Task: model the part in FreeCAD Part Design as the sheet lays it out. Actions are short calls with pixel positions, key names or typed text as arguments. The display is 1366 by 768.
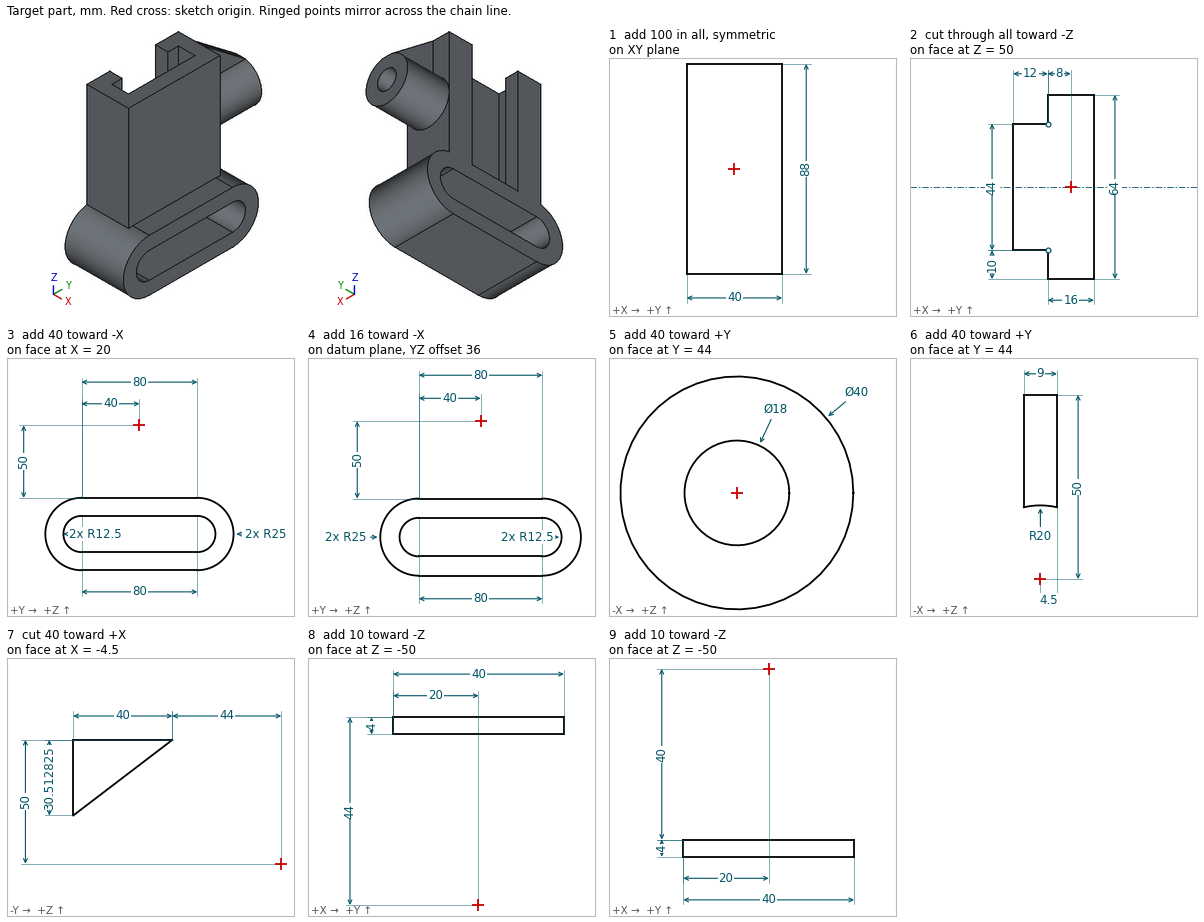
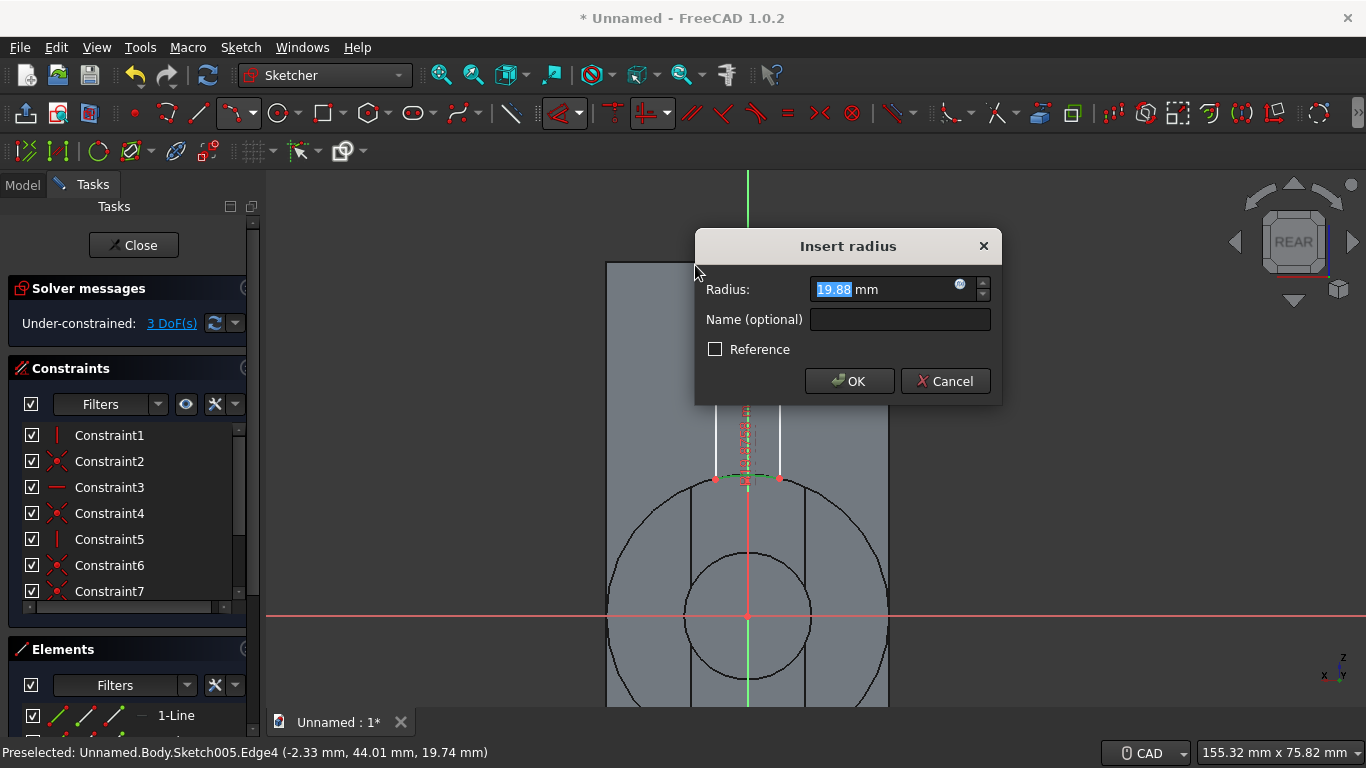
text(20)
key(Return)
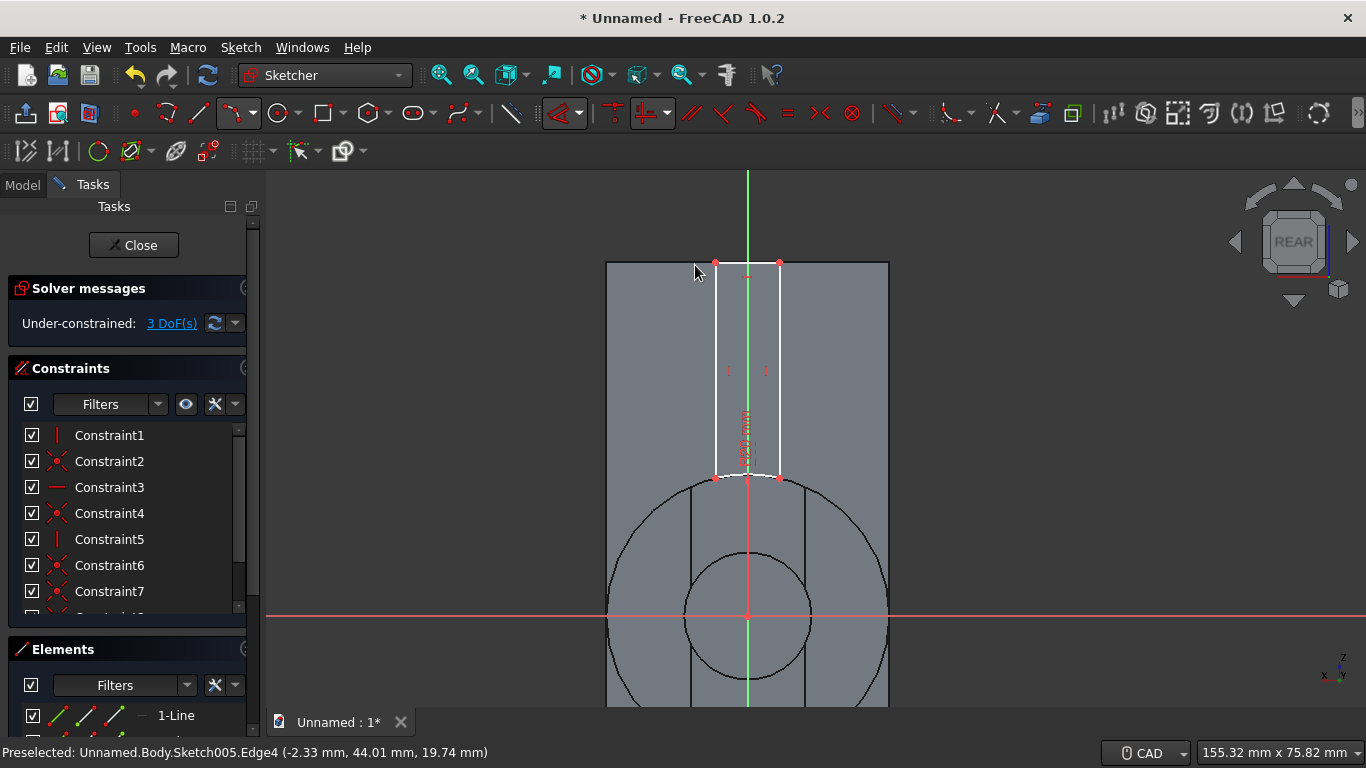
click(760, 263)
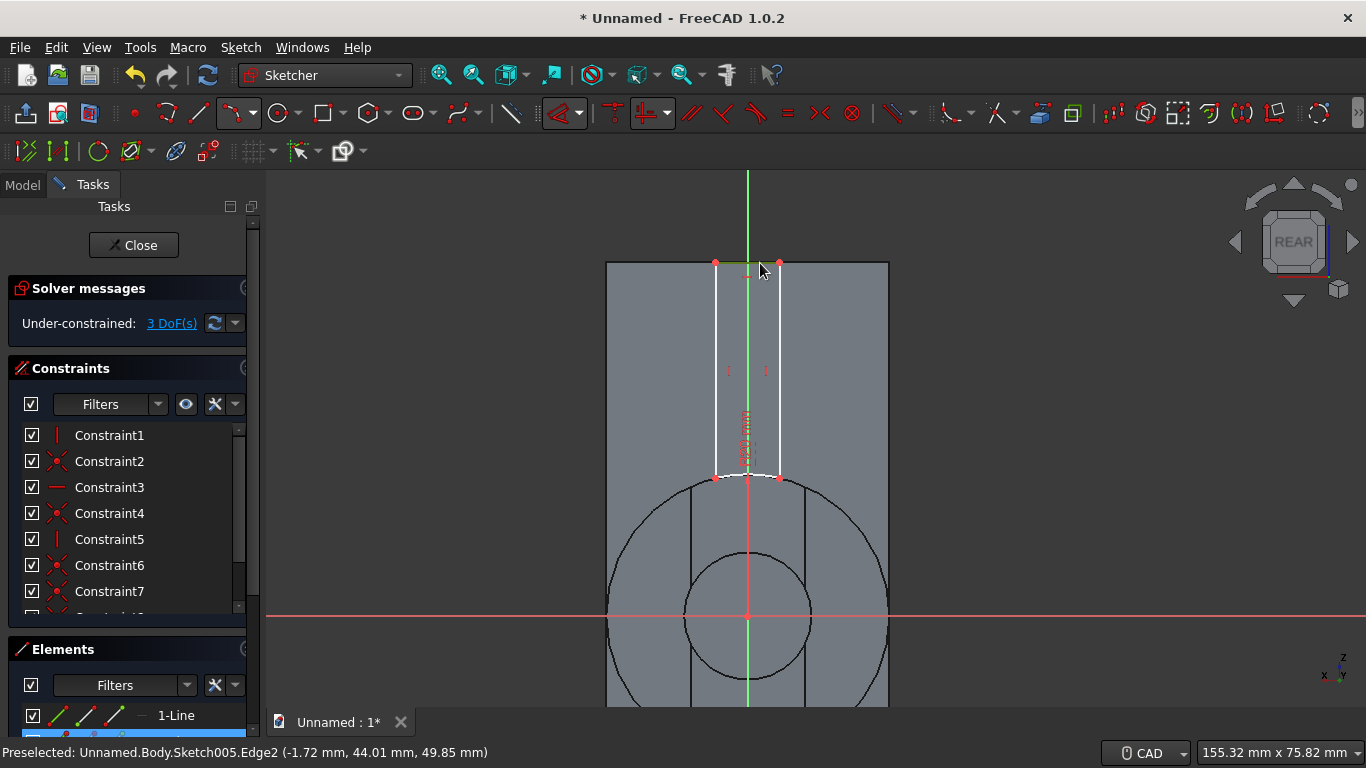
key(l)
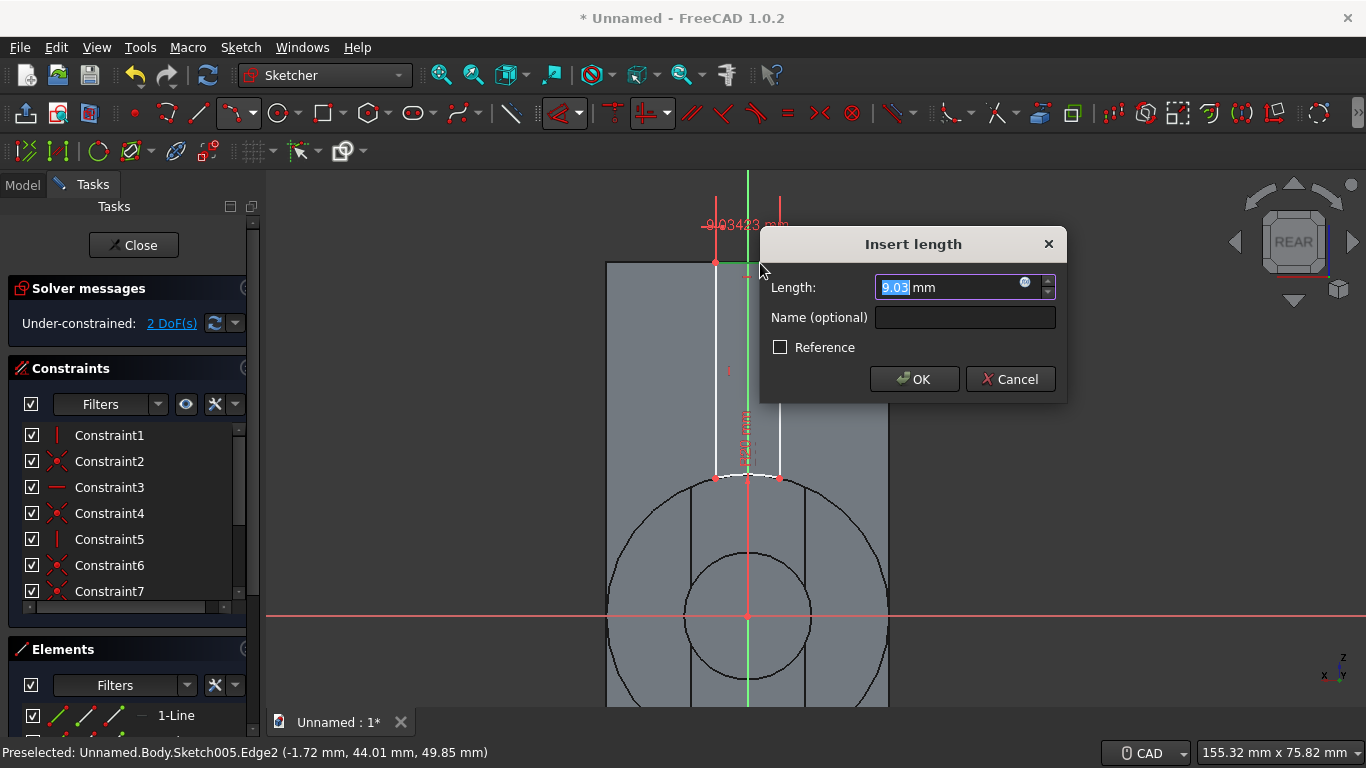
text(9)
key(Return)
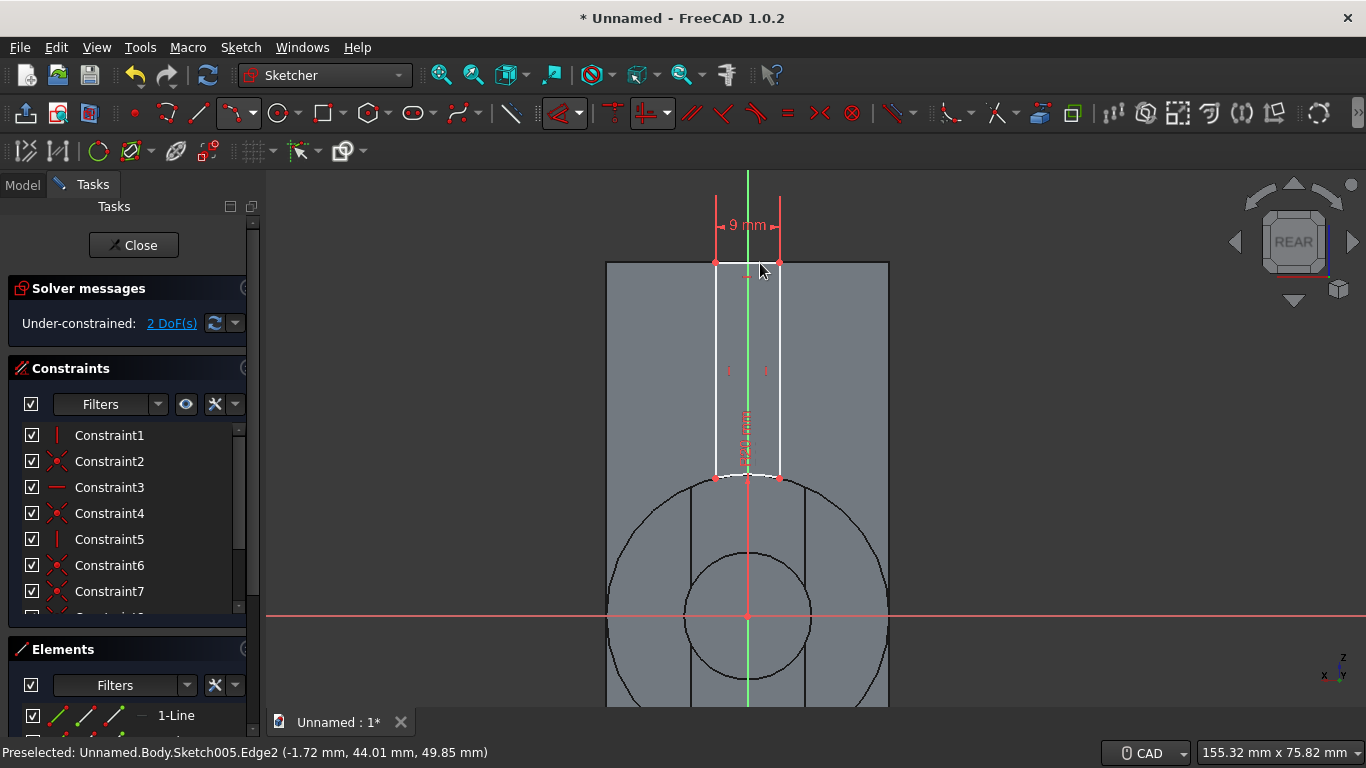
click(780, 263)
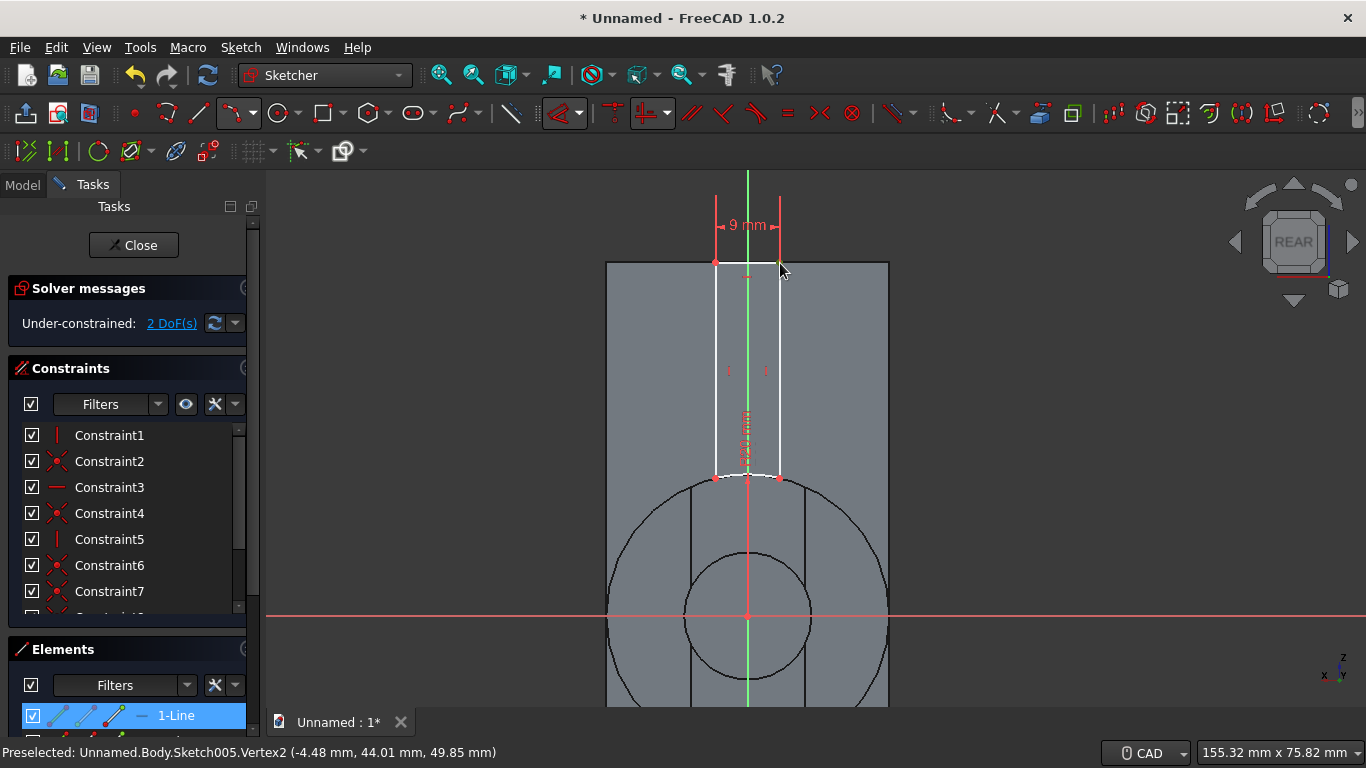
key(i)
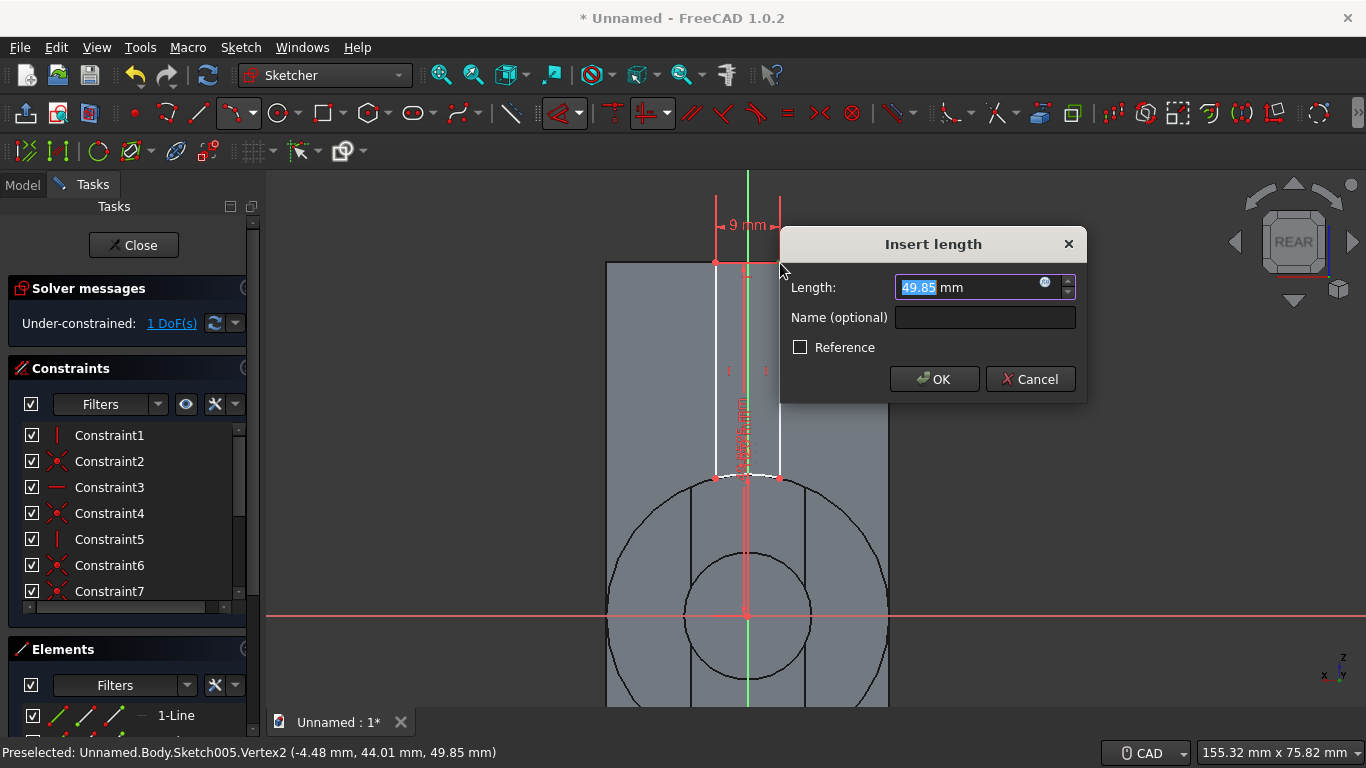
text(50)
key(Return)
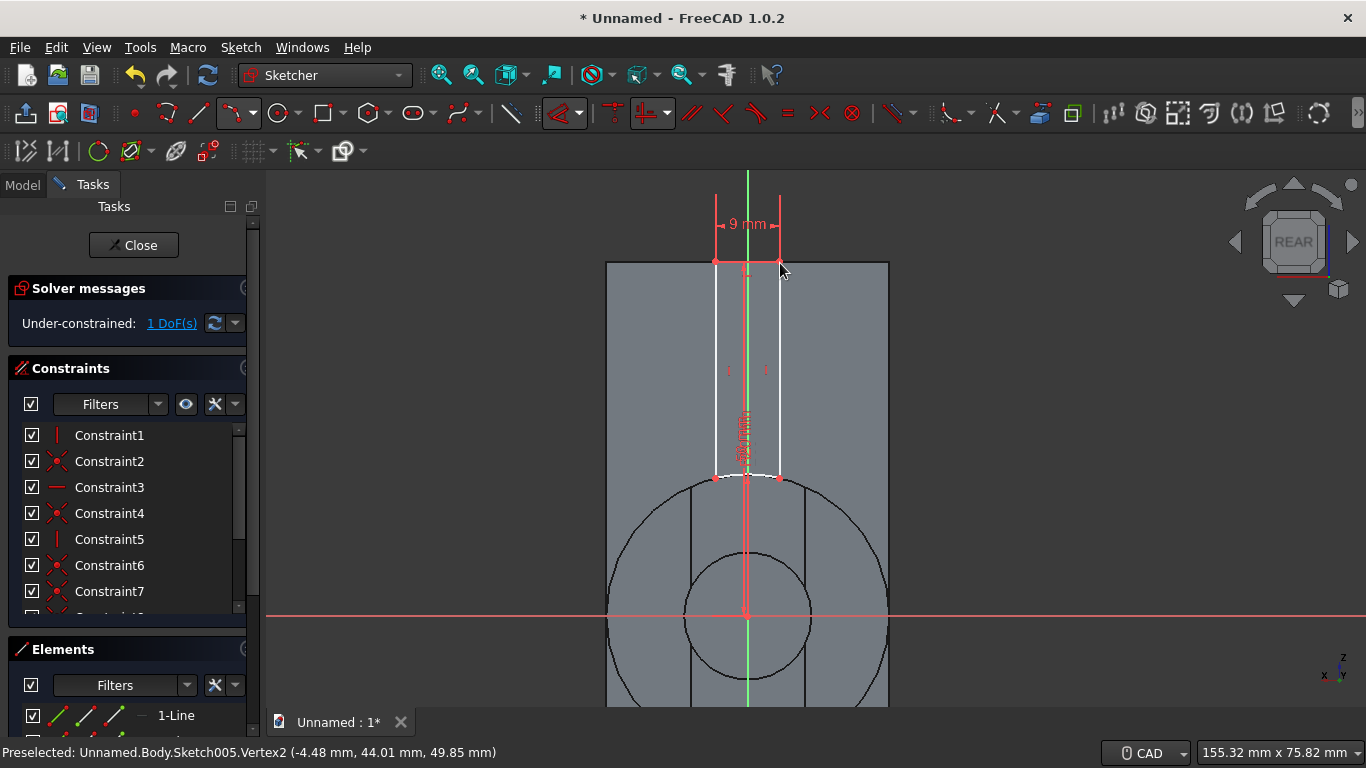
scroll(780, 478, up, 2)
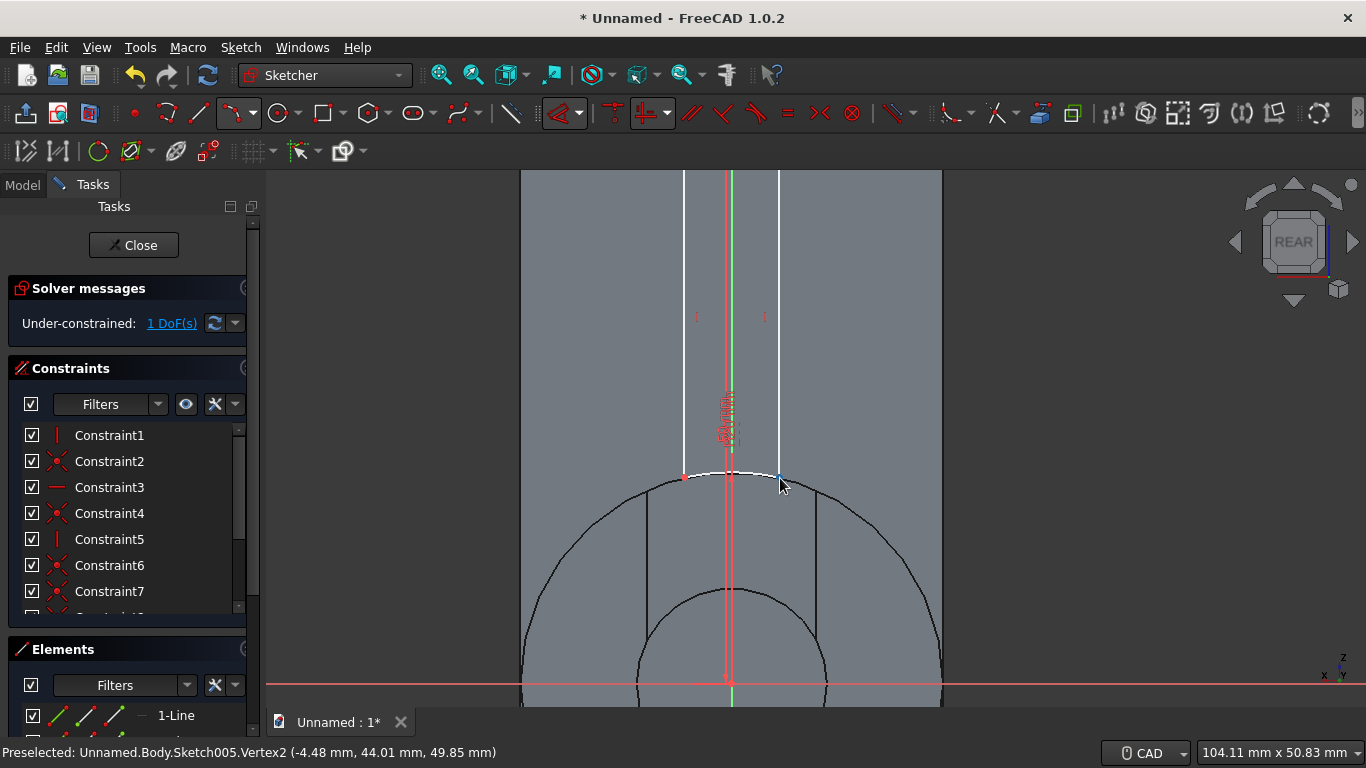
click(779, 478)